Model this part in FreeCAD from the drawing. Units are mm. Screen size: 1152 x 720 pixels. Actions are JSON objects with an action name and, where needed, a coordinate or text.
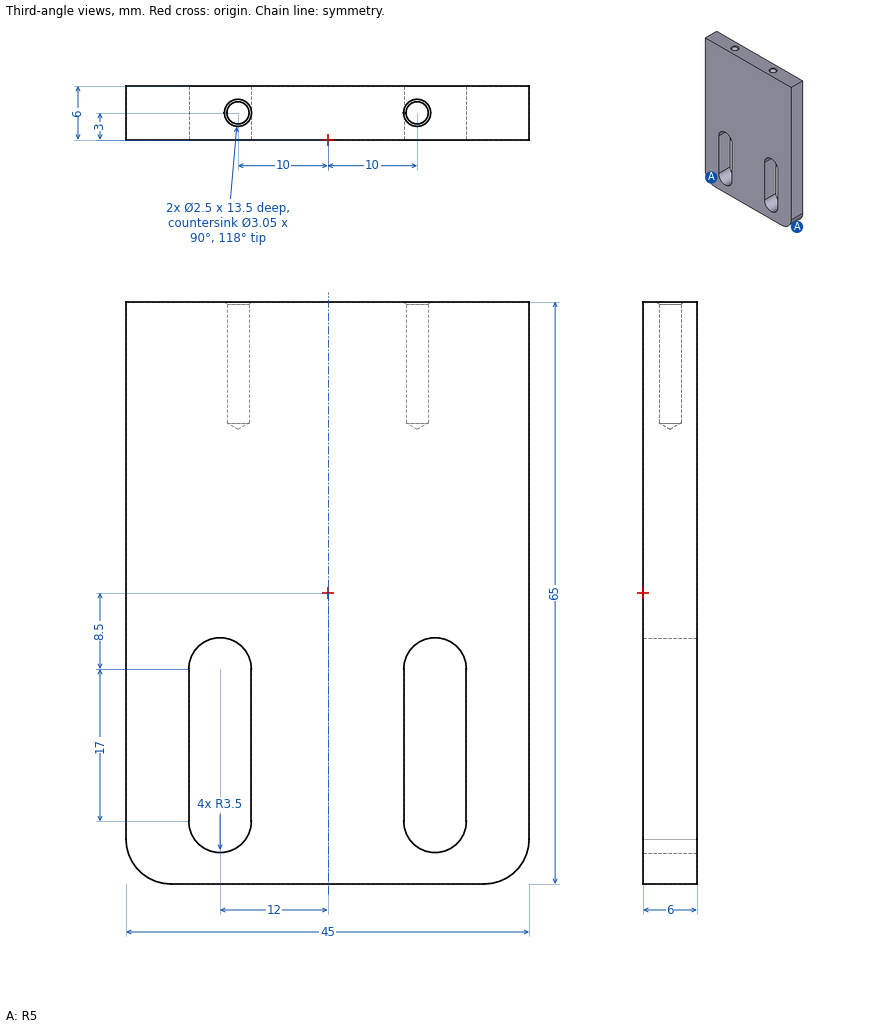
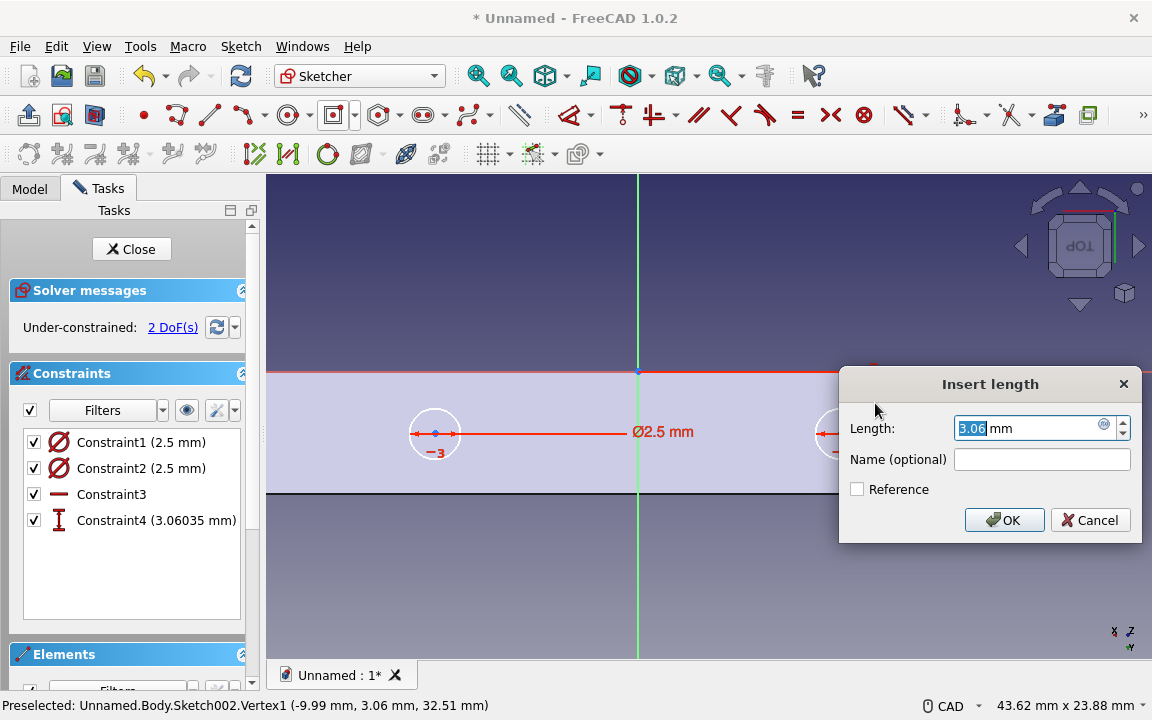
{"action": "type", "text": "3"}
{"action": "key", "text": "Return"}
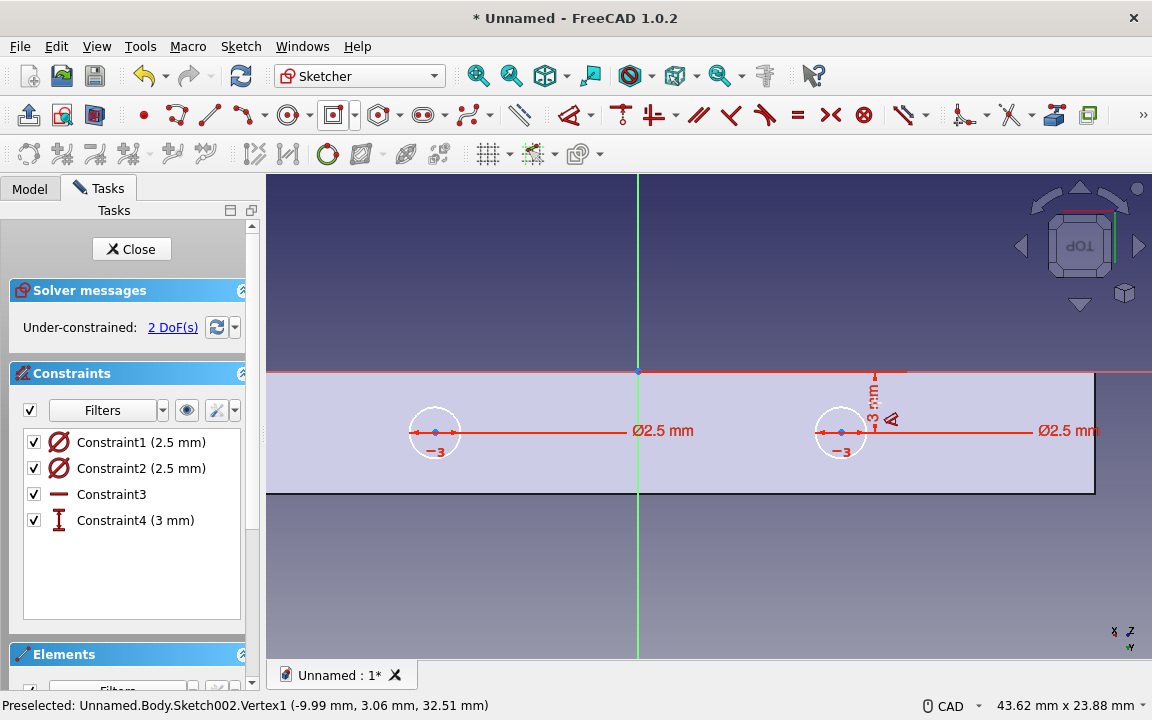
{"action": "left_click", "coordinate": [841, 433]}
{"action": "left_click", "coordinate": [740, 338]}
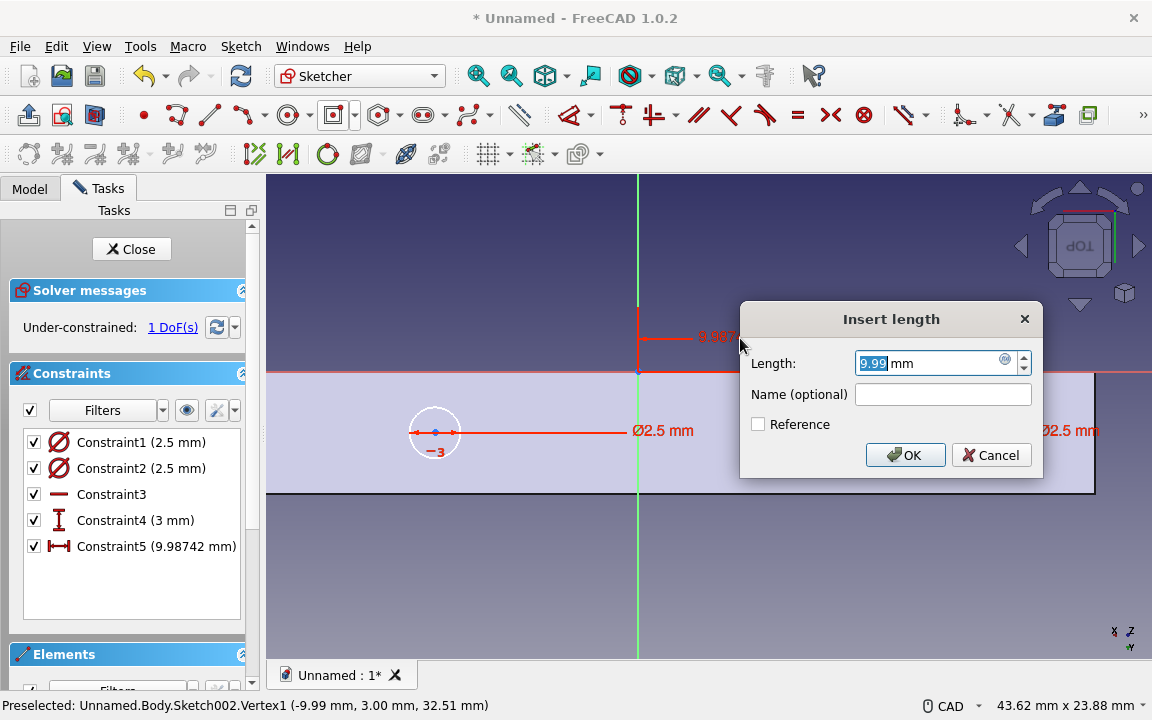
{"action": "type", "text": "10"}
{"action": "key", "text": "Return"}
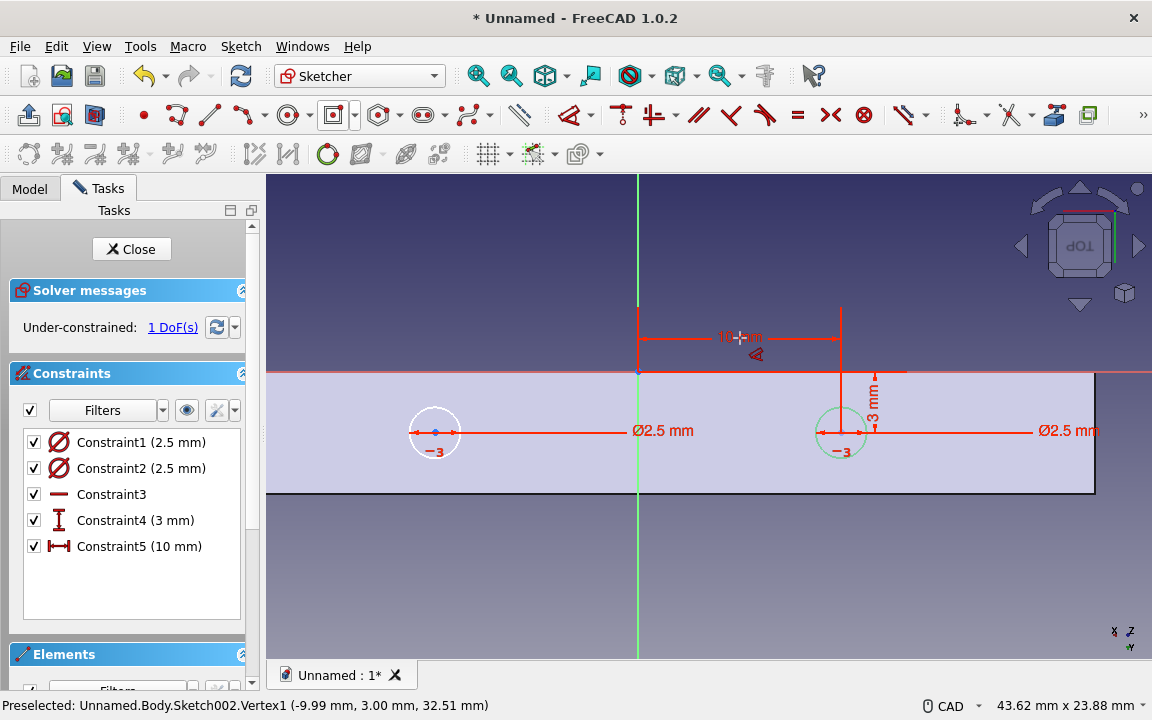
{"action": "left_click", "coordinate": [435, 433]}
{"action": "left_click", "coordinate": [537, 338]}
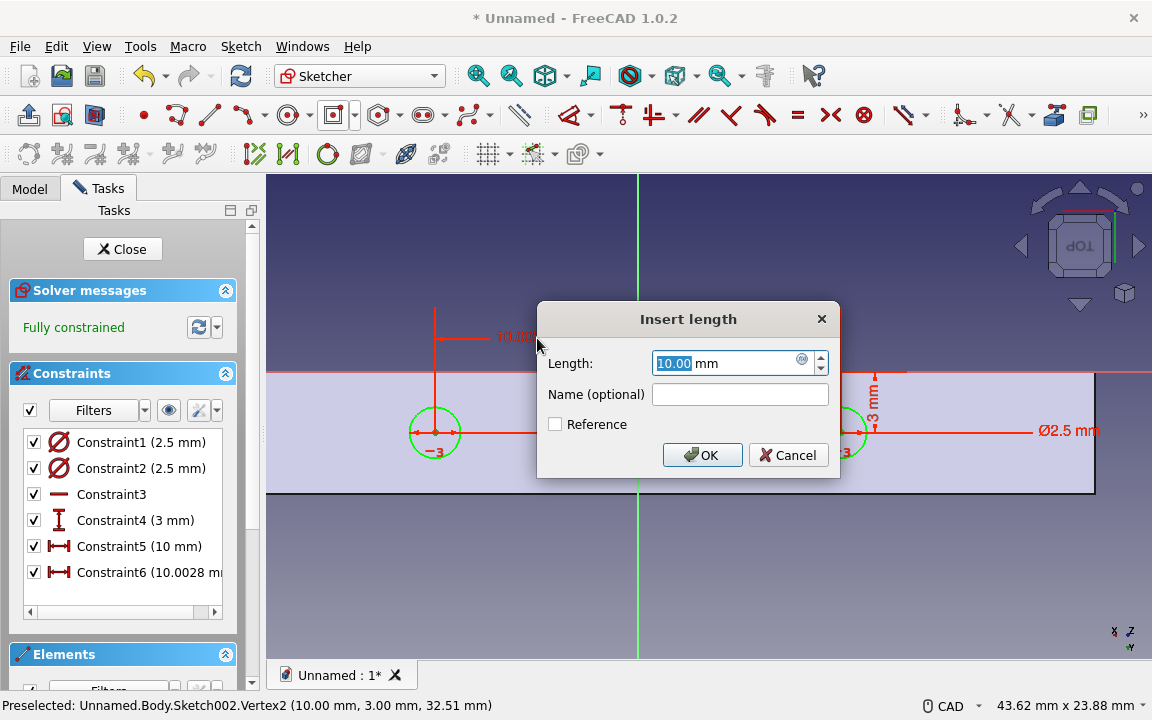
{"action": "type", "text": "10"}
{"action": "key", "text": "Return"}
{"action": "key", "text": "Escape"}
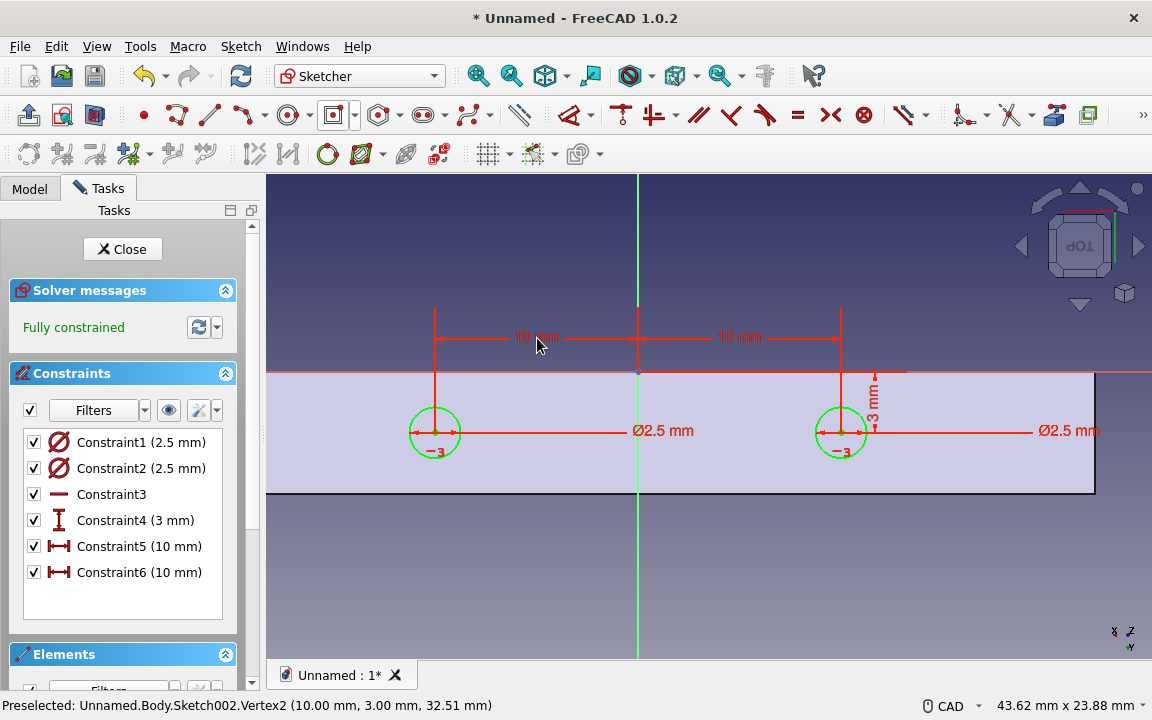
{"action": "left_click", "coordinate": [123, 249]}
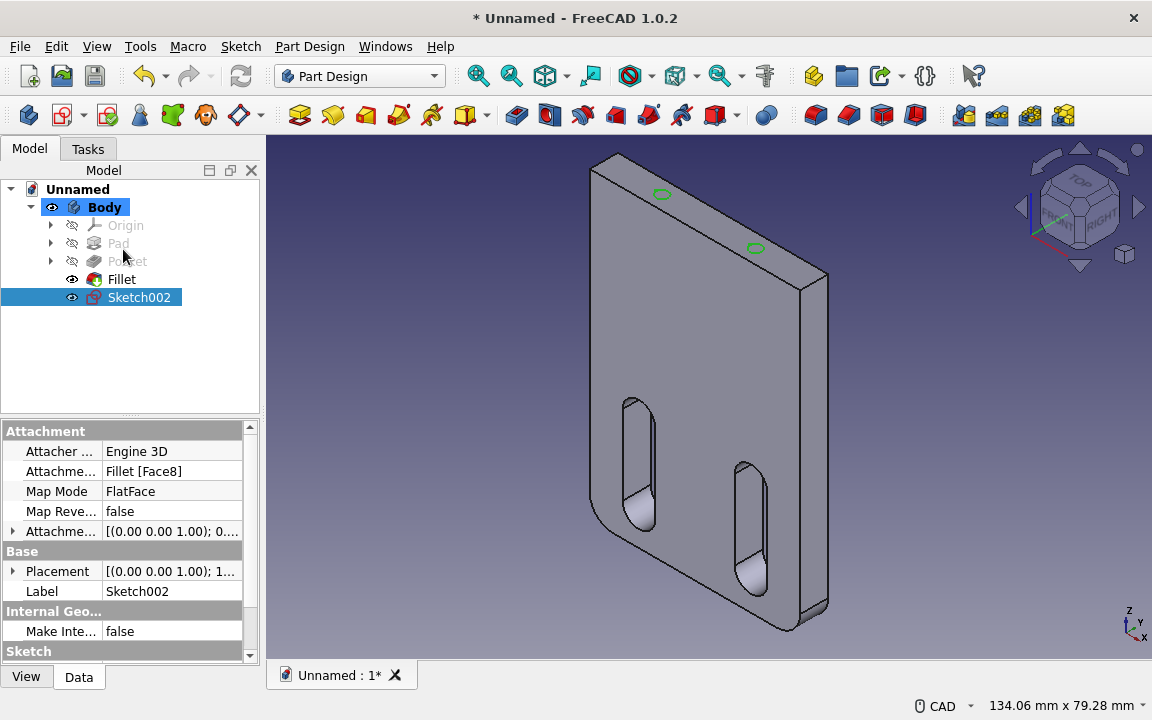
{"action": "left_click", "coordinate": [550, 116]}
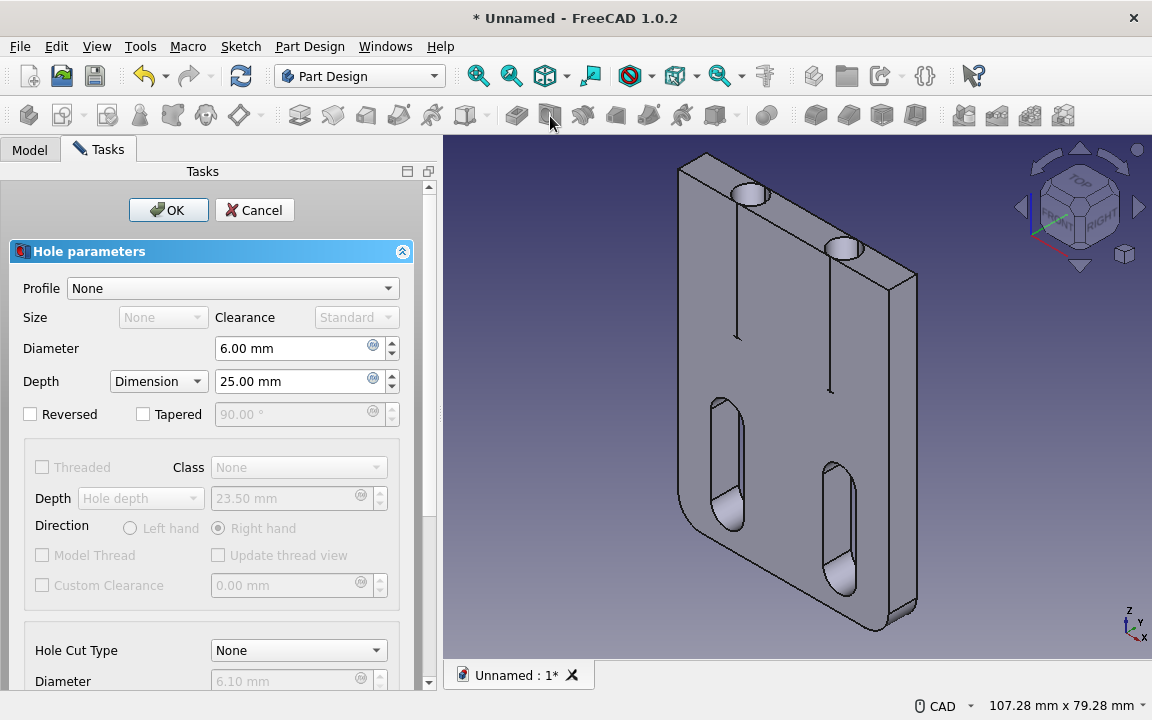
{"action": "triple_click", "coordinate": [300, 348]}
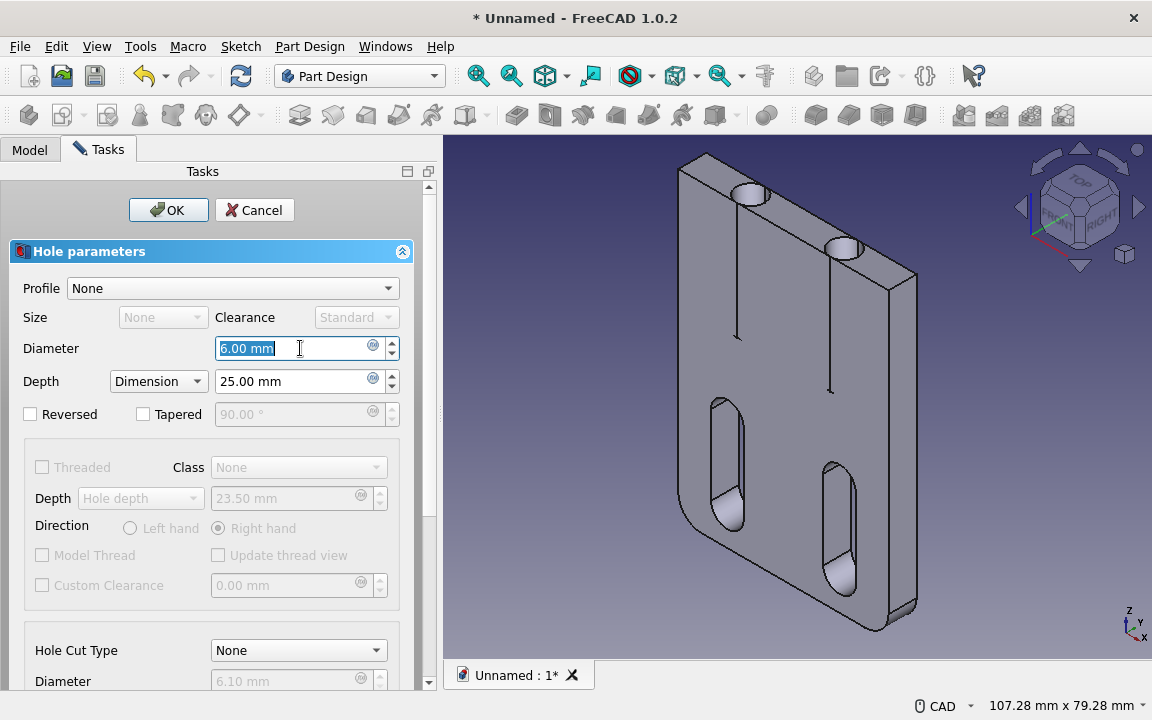
{"action": "type", "text": "2.5"}
{"action": "key", "text": "Tab"}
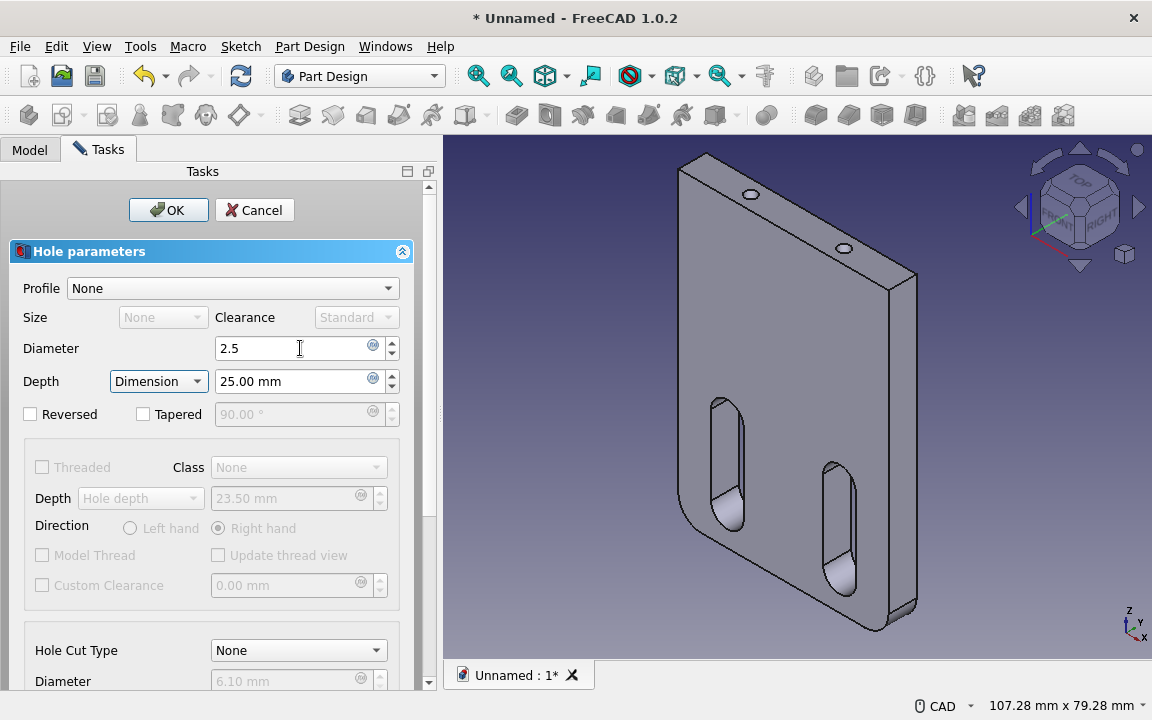
{"action": "triple_click", "coordinate": [300, 382]}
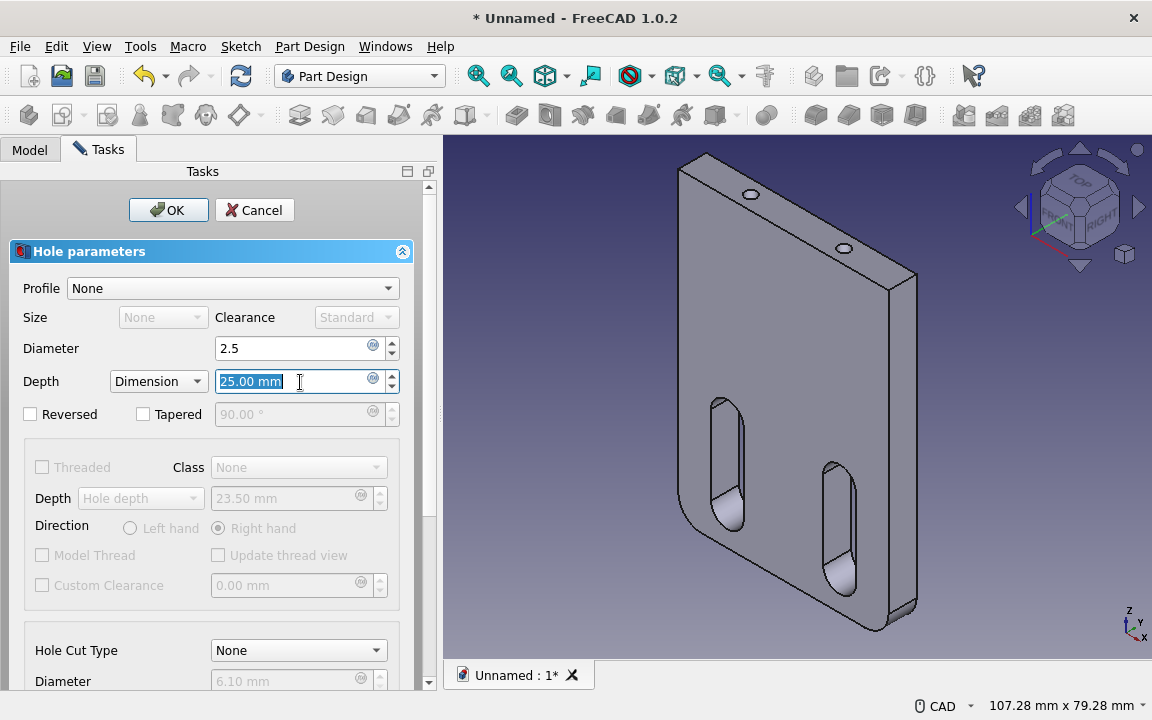
{"action": "type", "text": "13.5"}
{"action": "key", "text": "Tab"}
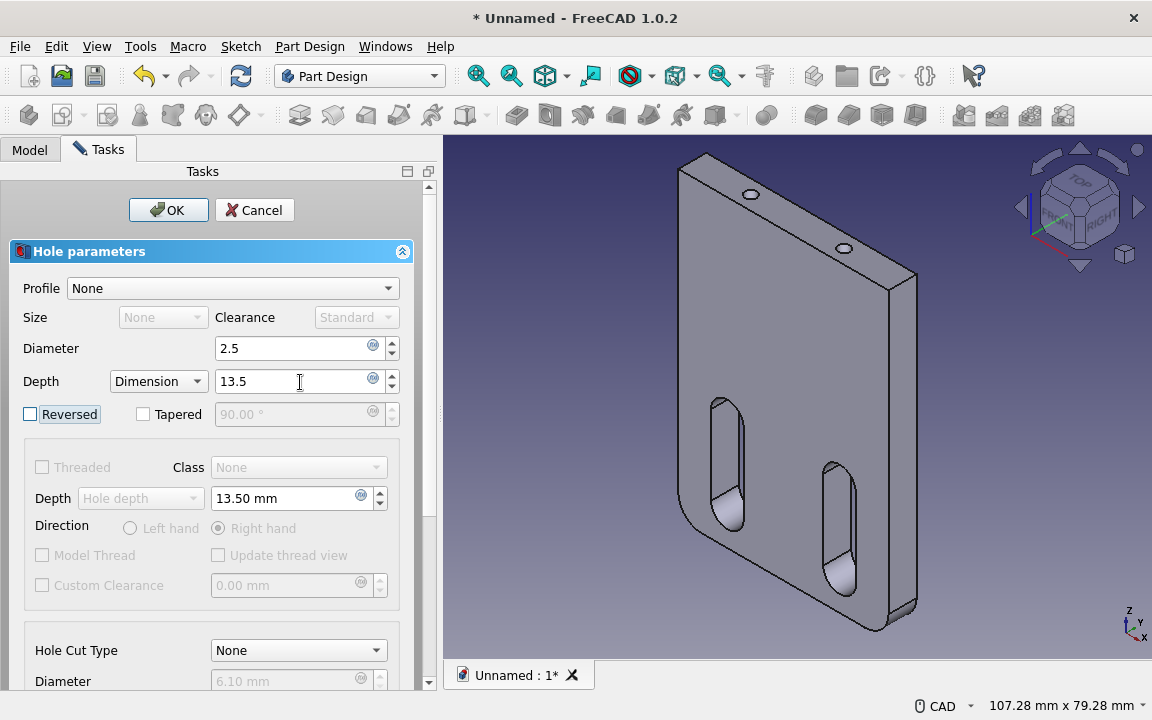
{"action": "left_click", "coordinate": [300, 650]}